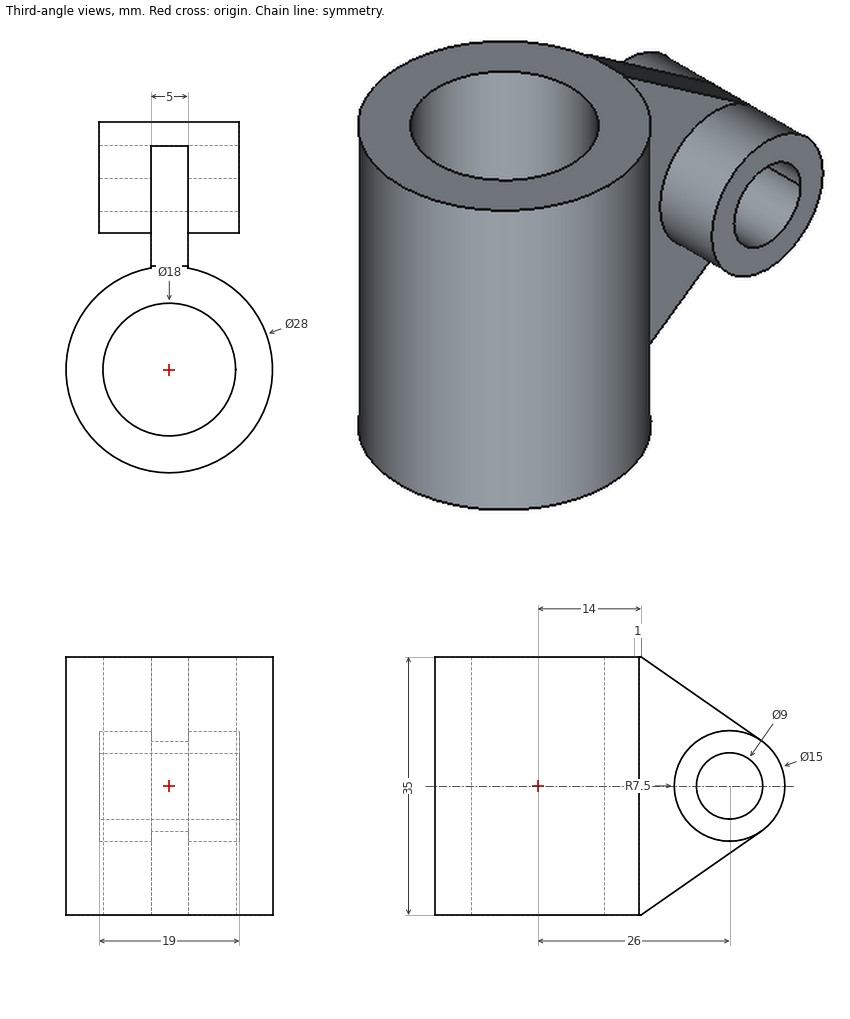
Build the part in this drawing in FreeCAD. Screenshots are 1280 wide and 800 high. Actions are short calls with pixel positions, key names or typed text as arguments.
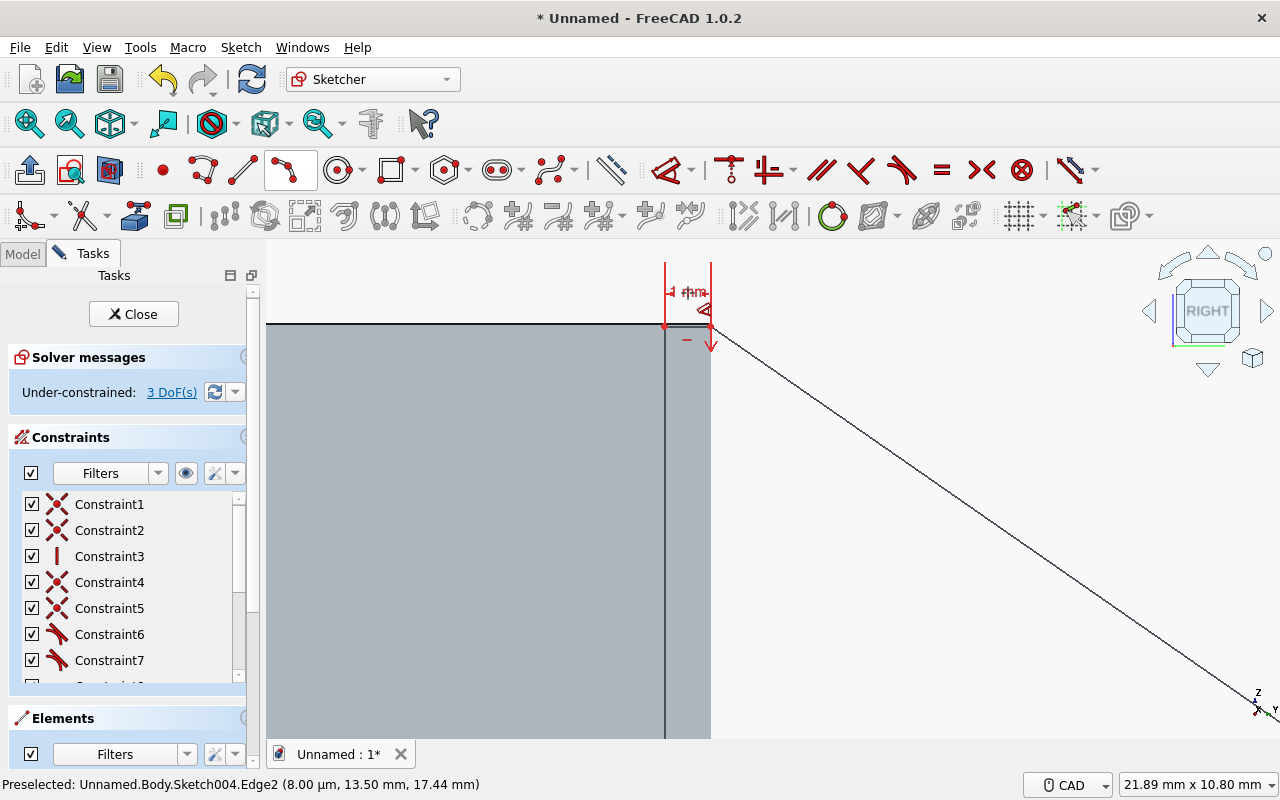
scroll(689, 326, down, 8)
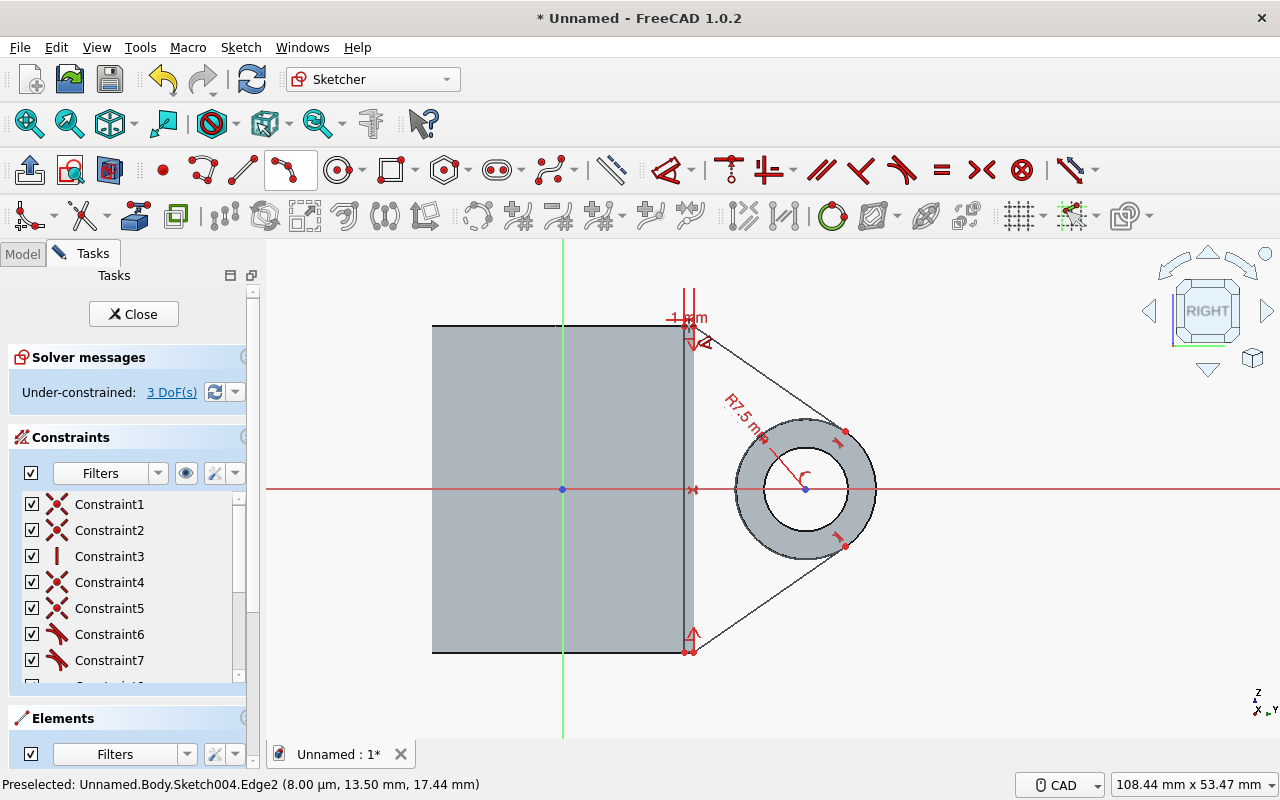
click(684, 392)
click(650, 414)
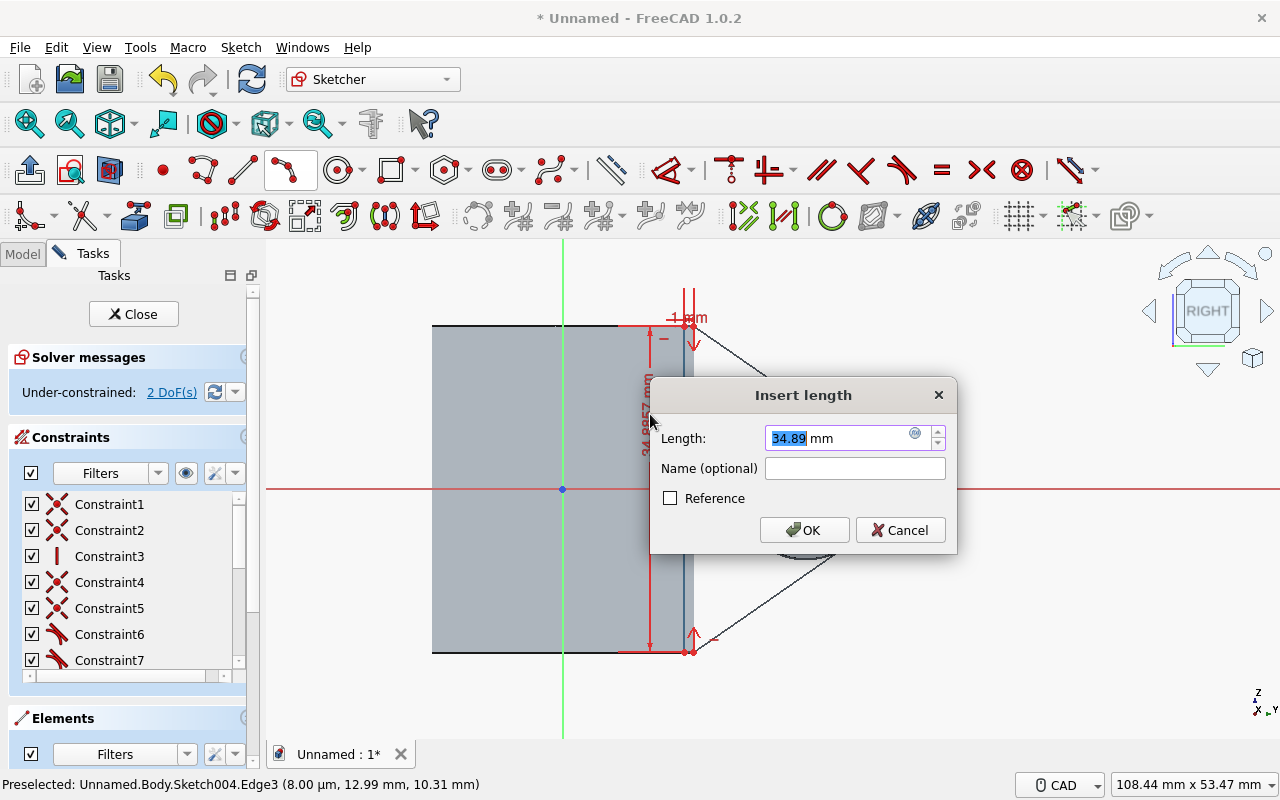
text(35)
key(Return)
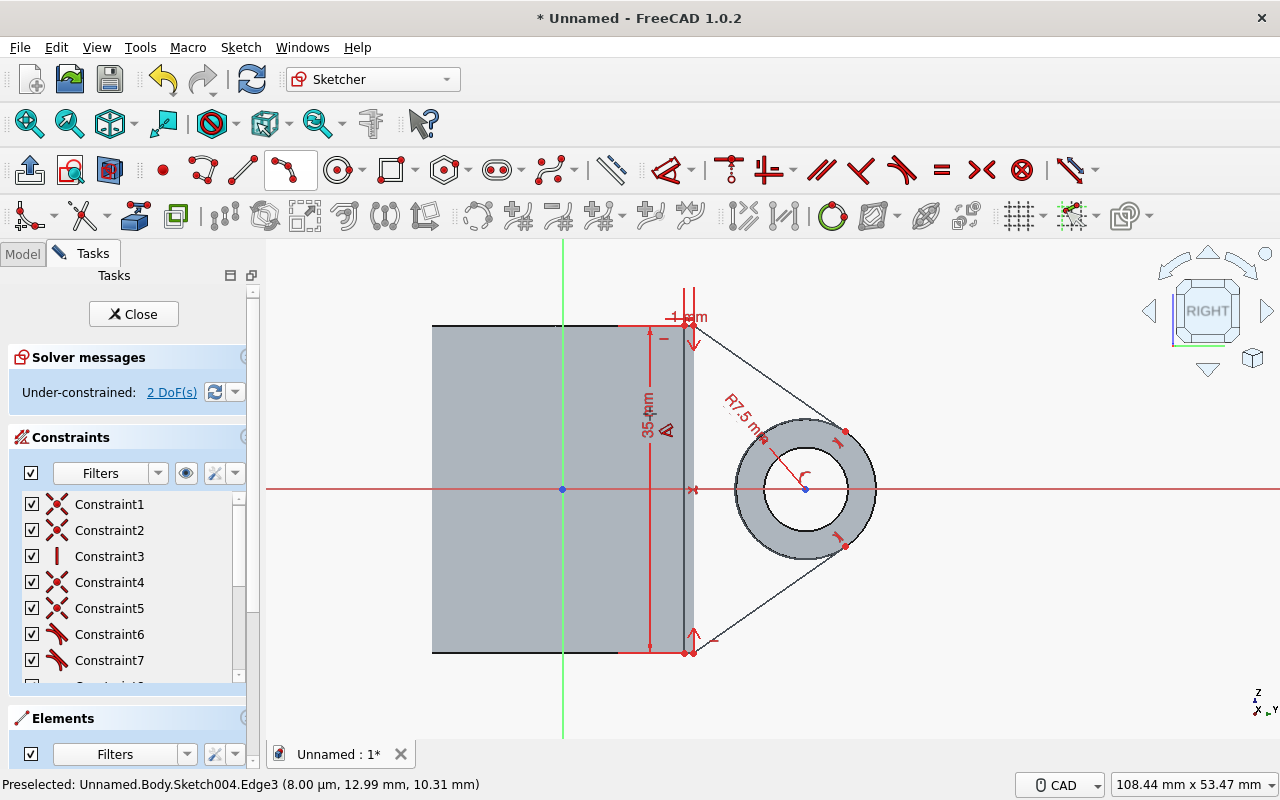
scroll(694, 326, up, 2)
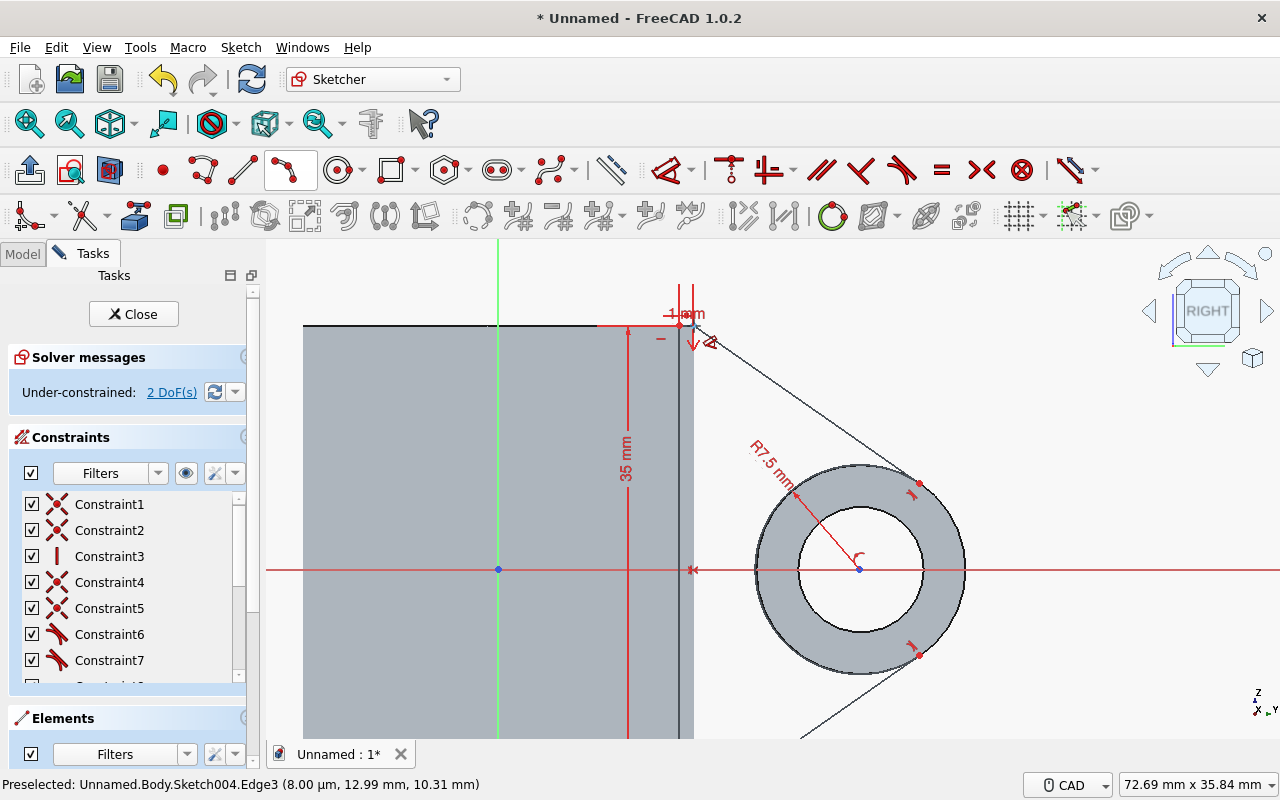
click(693, 326)
click(596, 292)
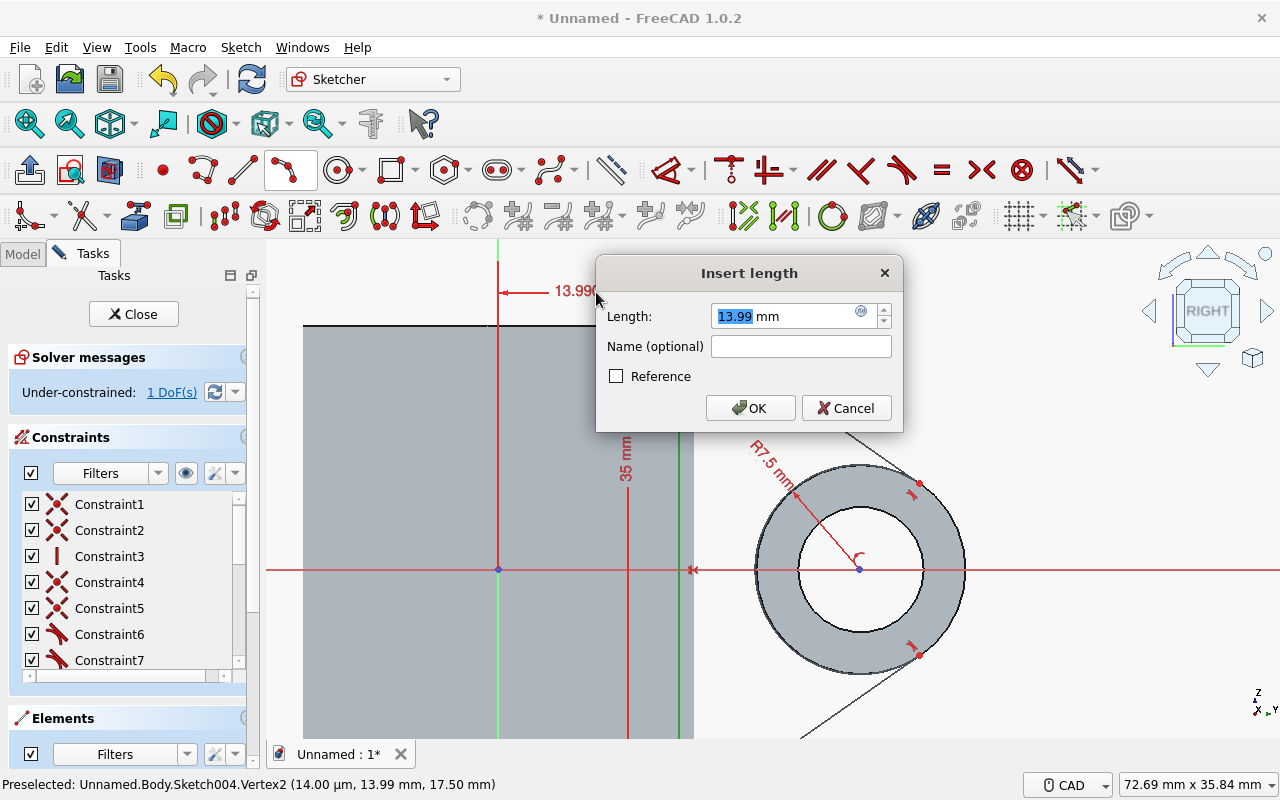
text(14)
key(Return)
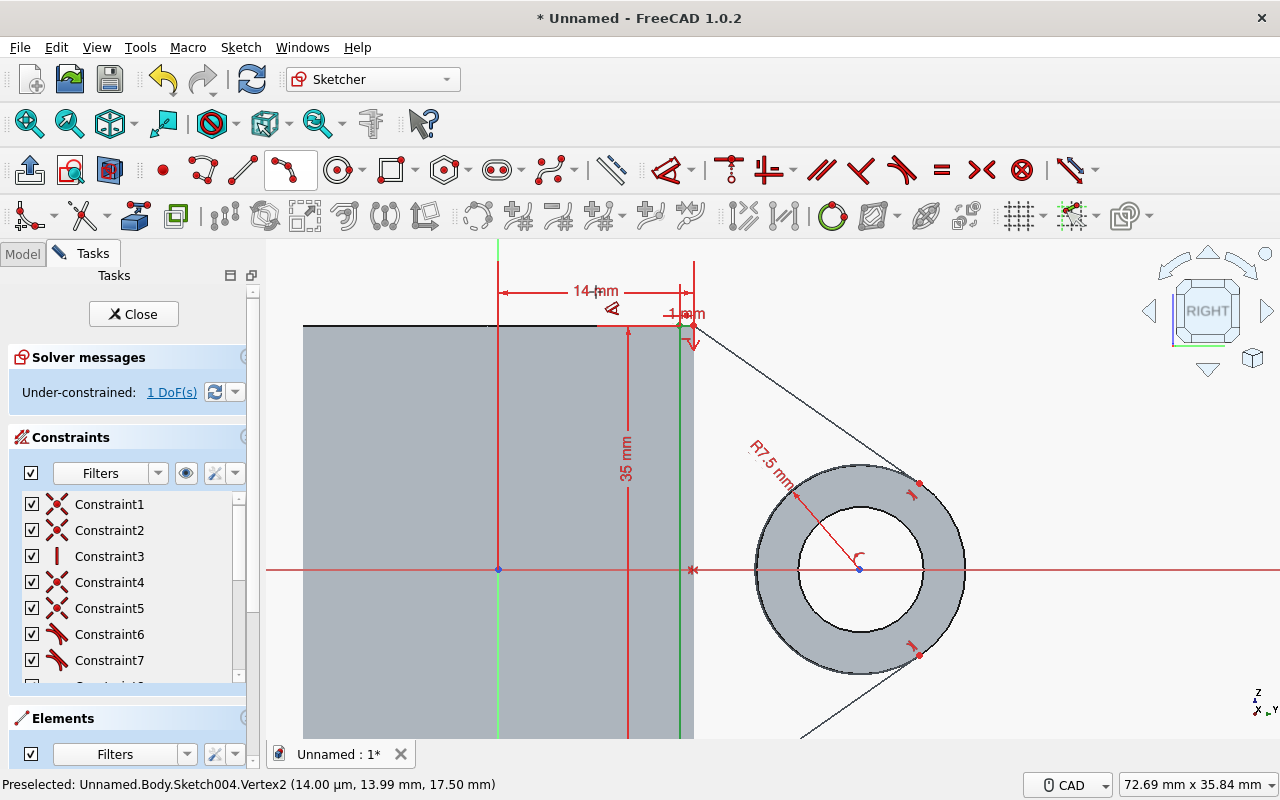
click(860, 570)
click(596, 604)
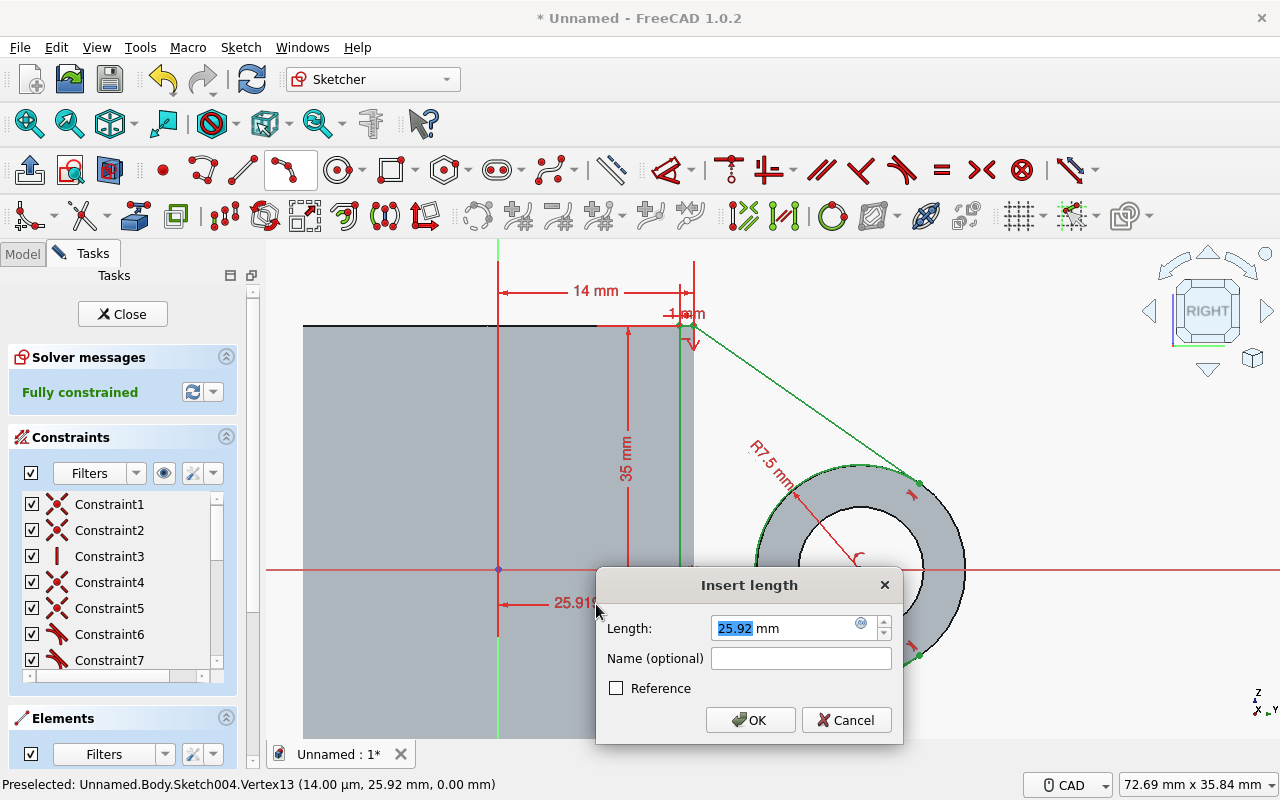
text(26)
key(Return)
key(Escape)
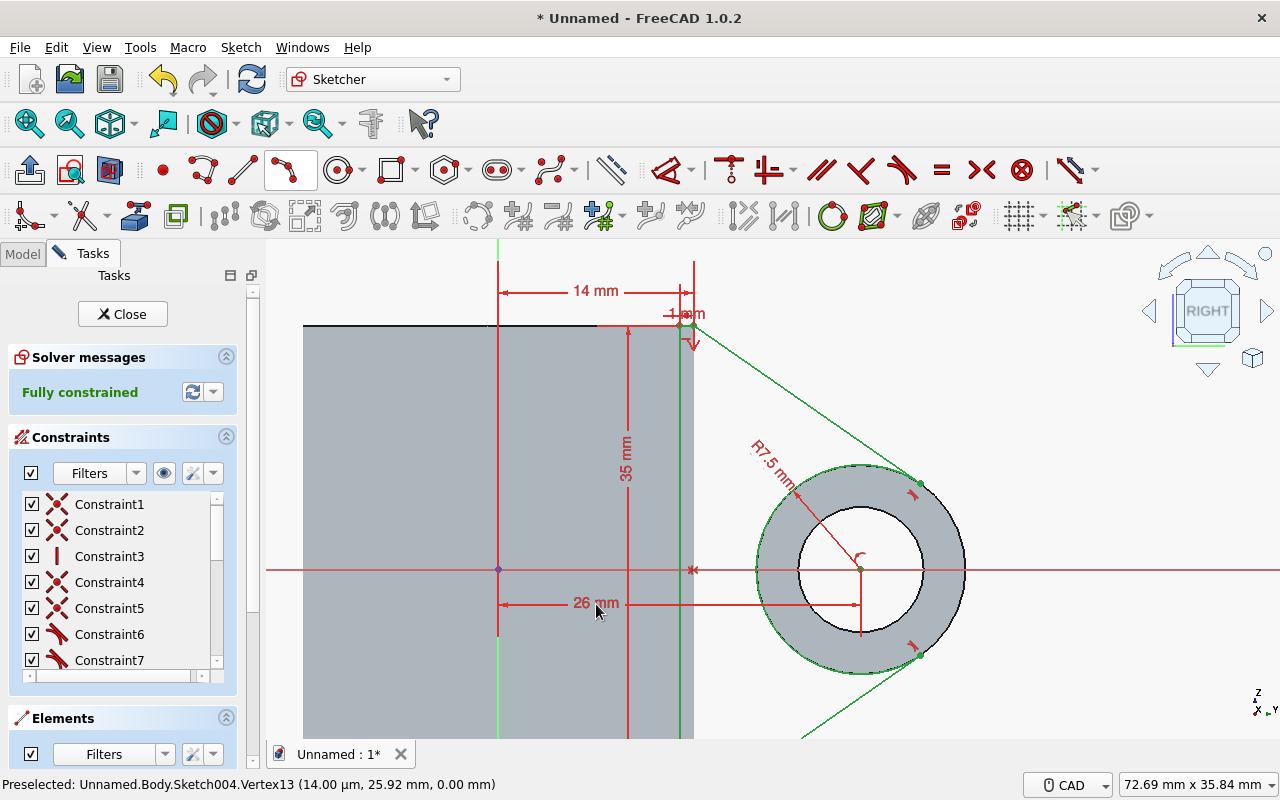
click(123, 314)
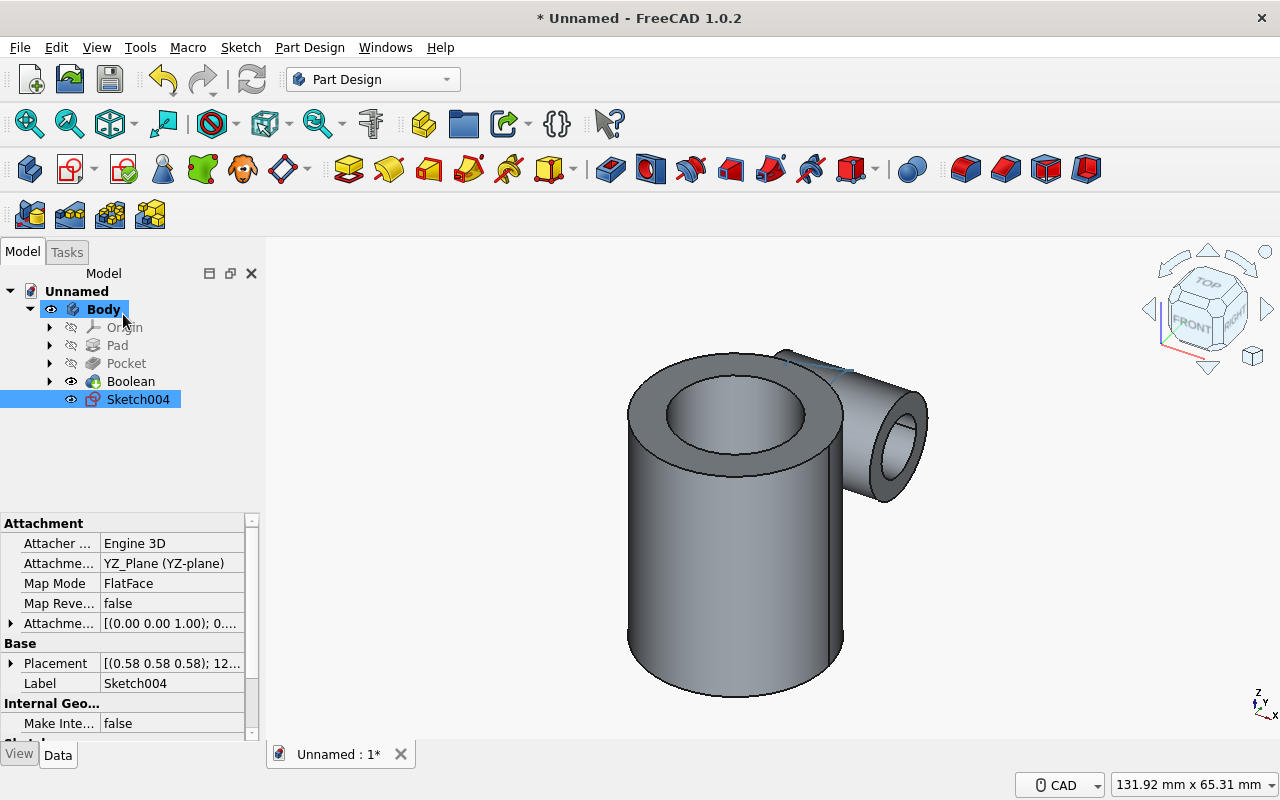
click(350, 170)